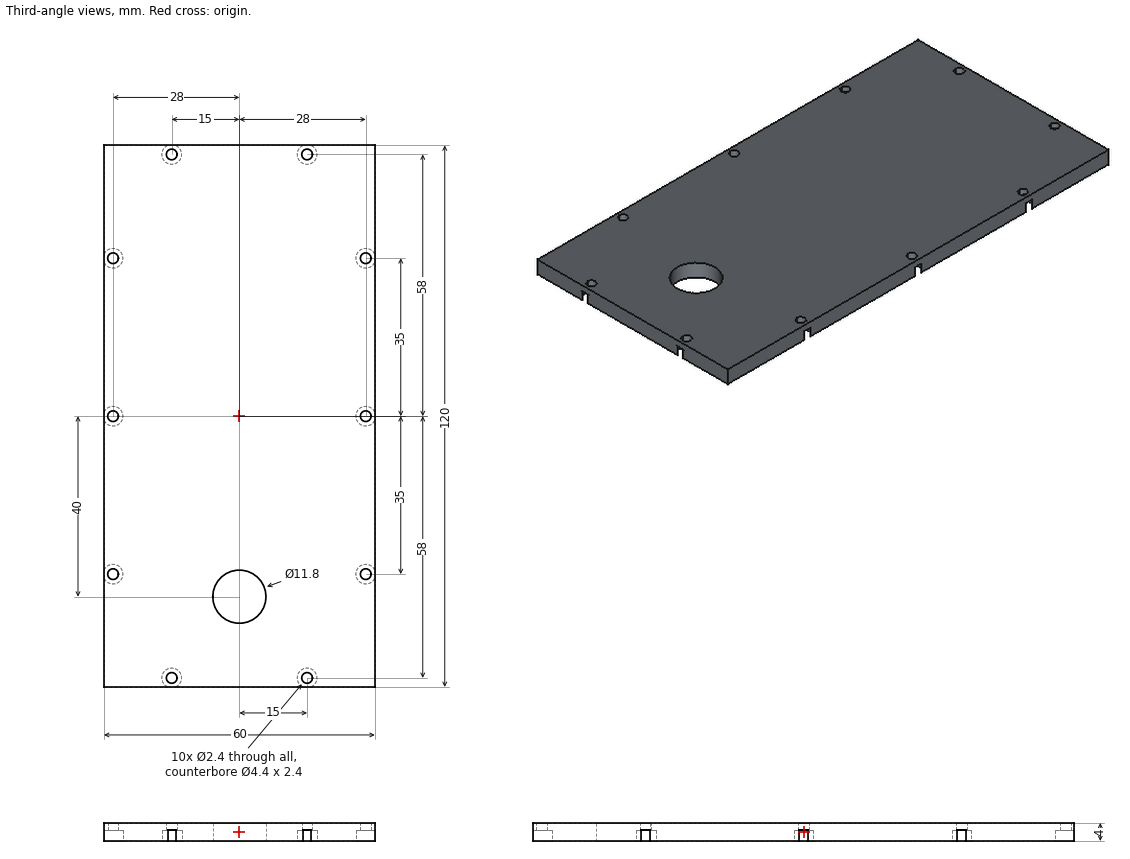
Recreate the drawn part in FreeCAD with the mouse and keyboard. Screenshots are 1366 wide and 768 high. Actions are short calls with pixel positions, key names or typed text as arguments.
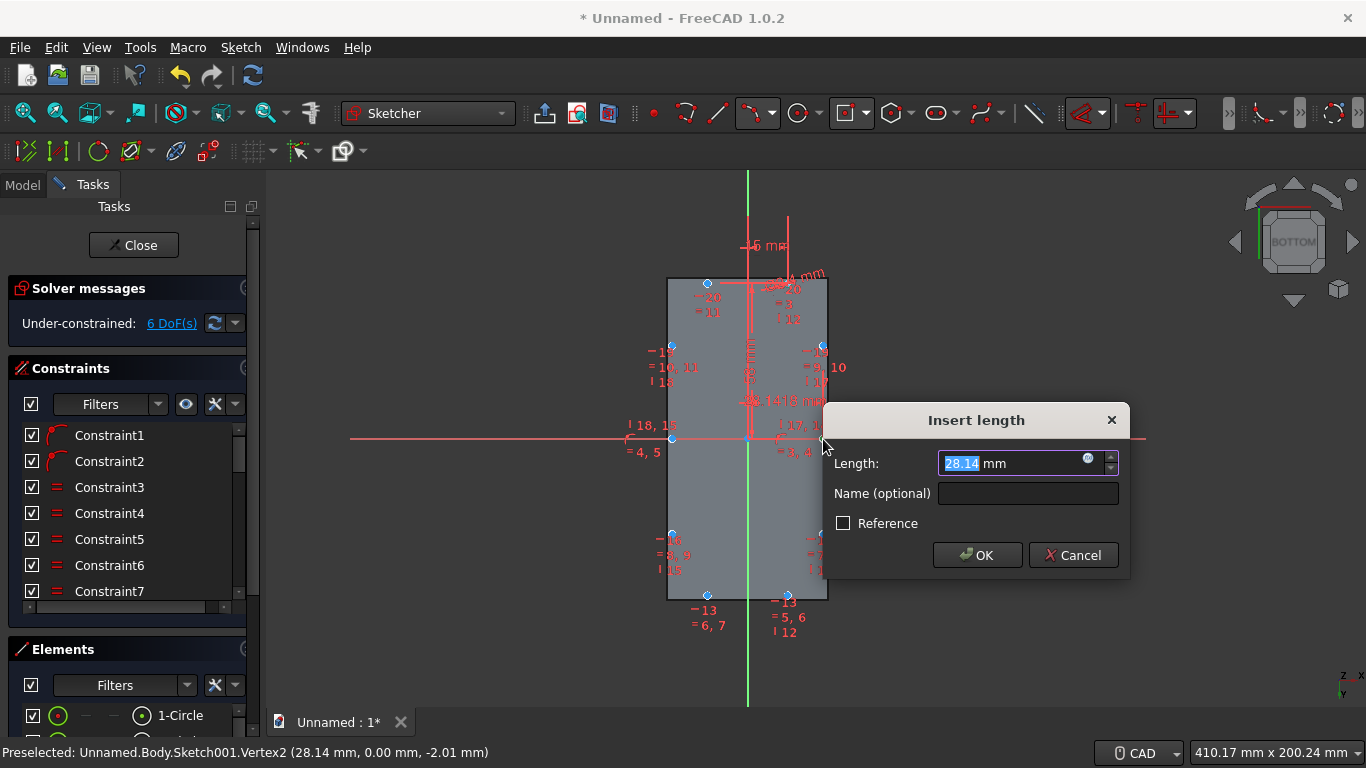
text(28)
key(Return)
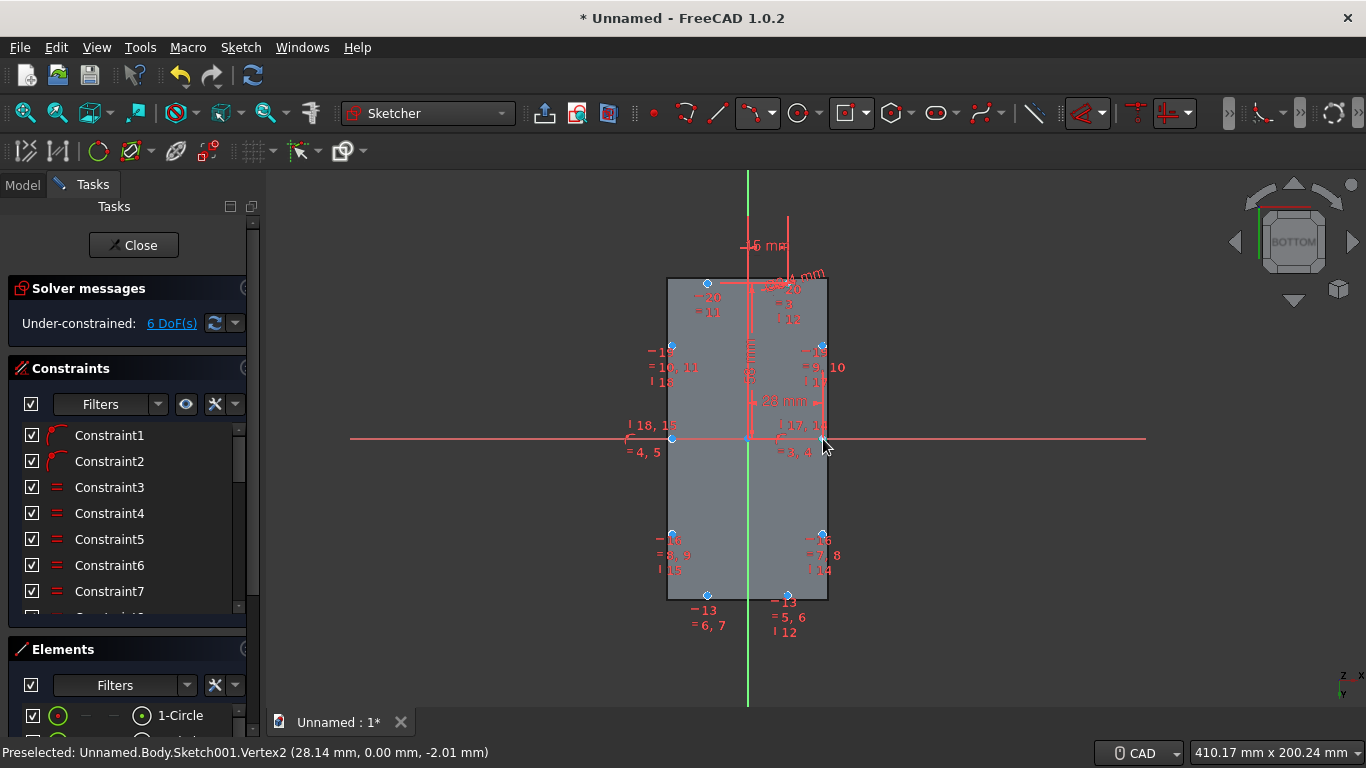
click(672, 439)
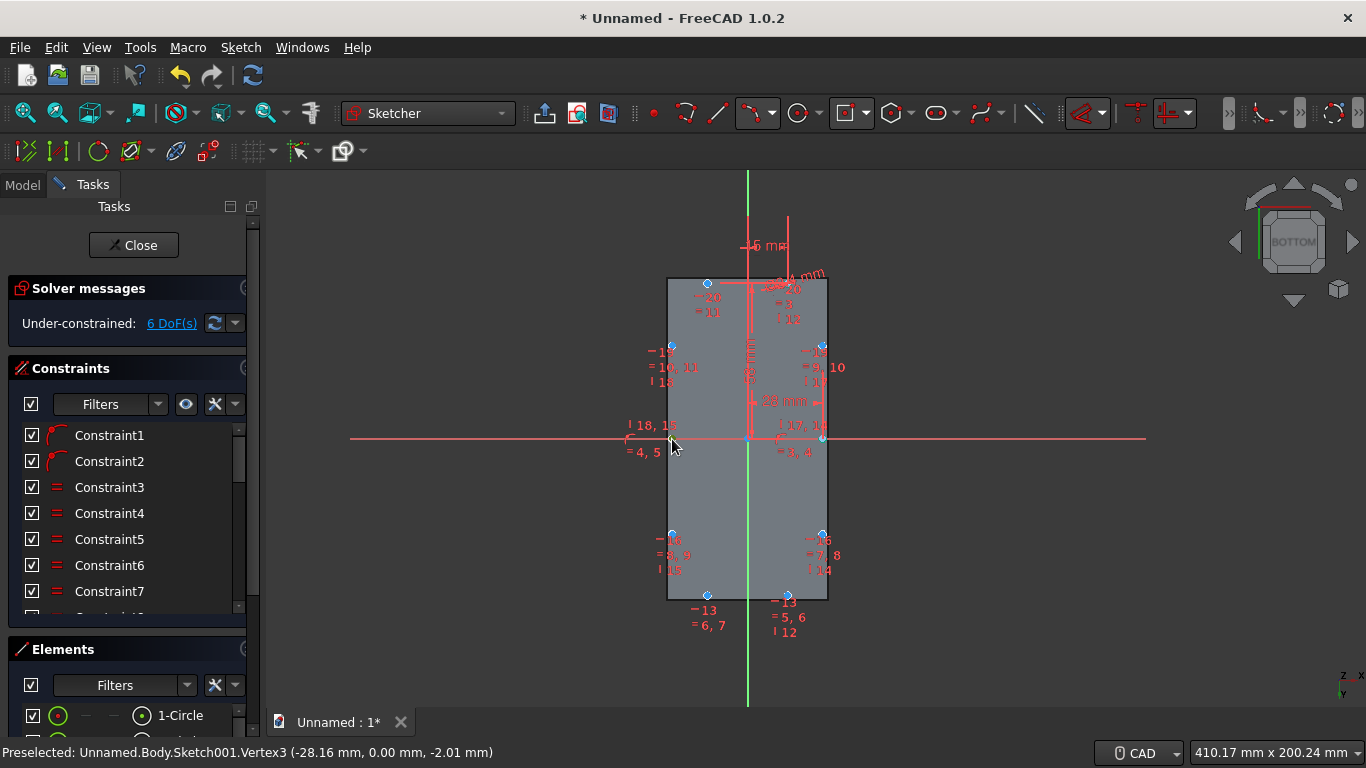
click(1104, 114)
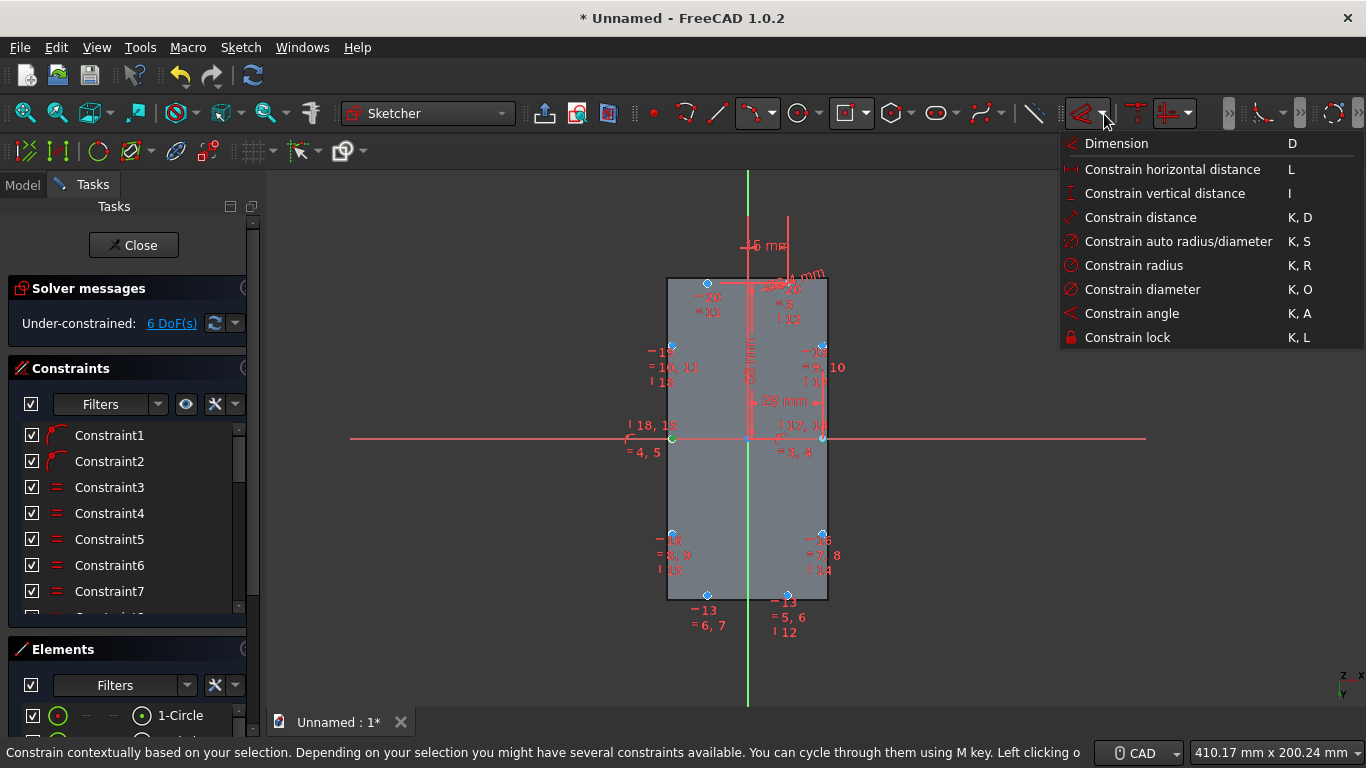
click(1212, 169)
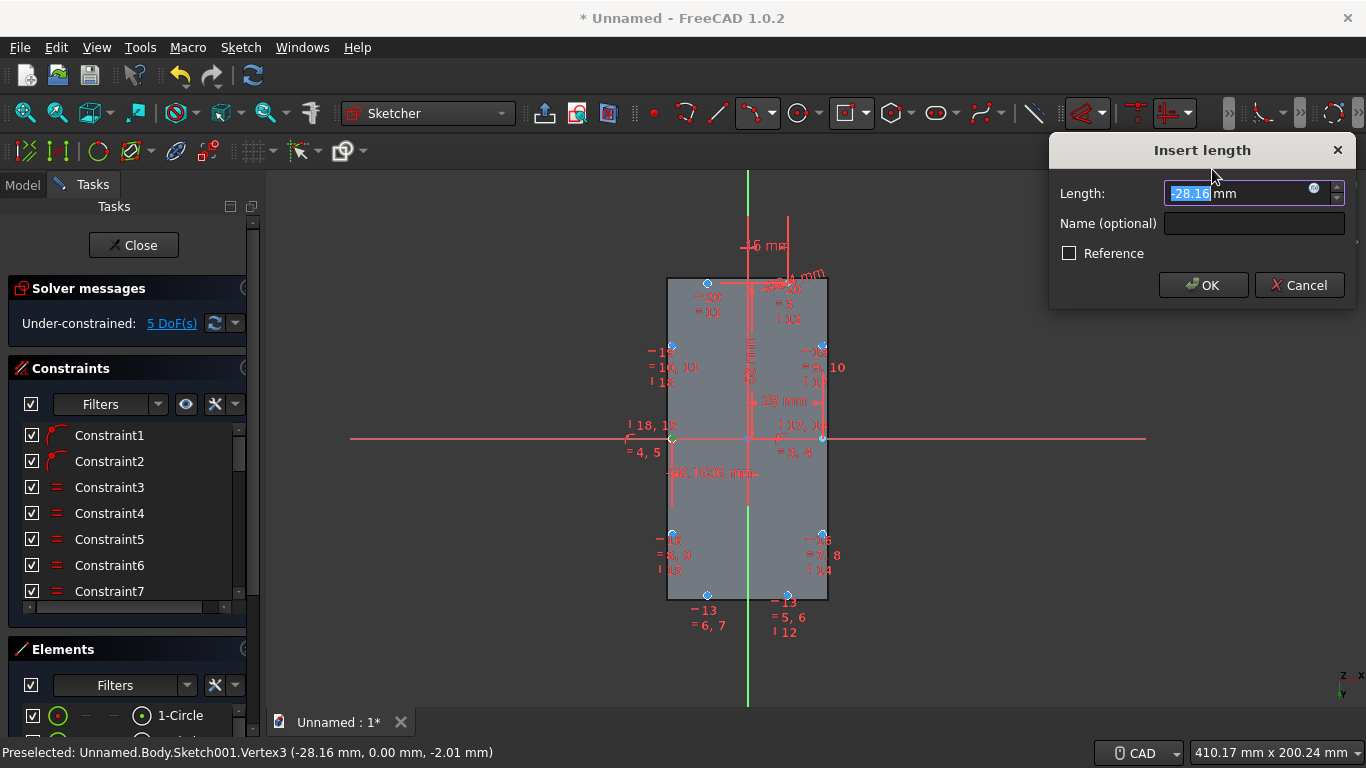
text(-28)
key(Return)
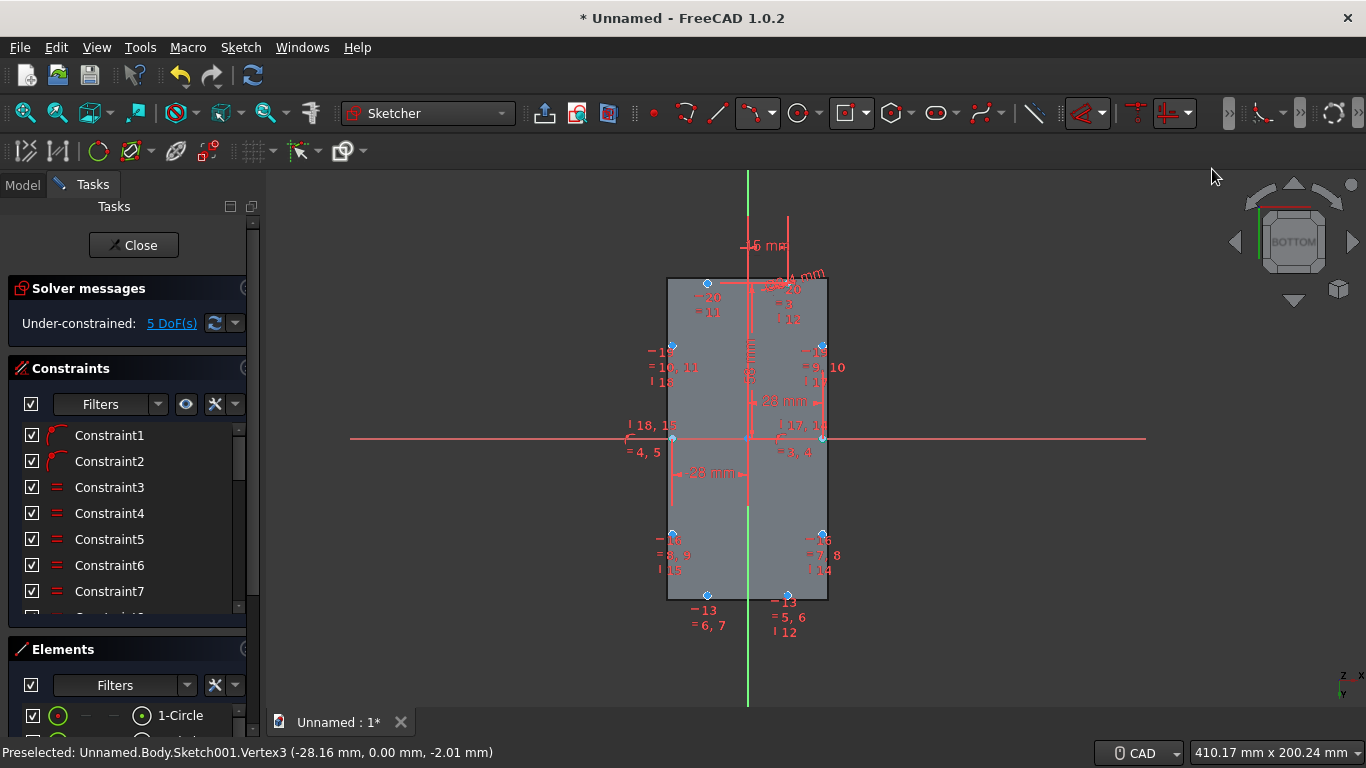
click(788, 596)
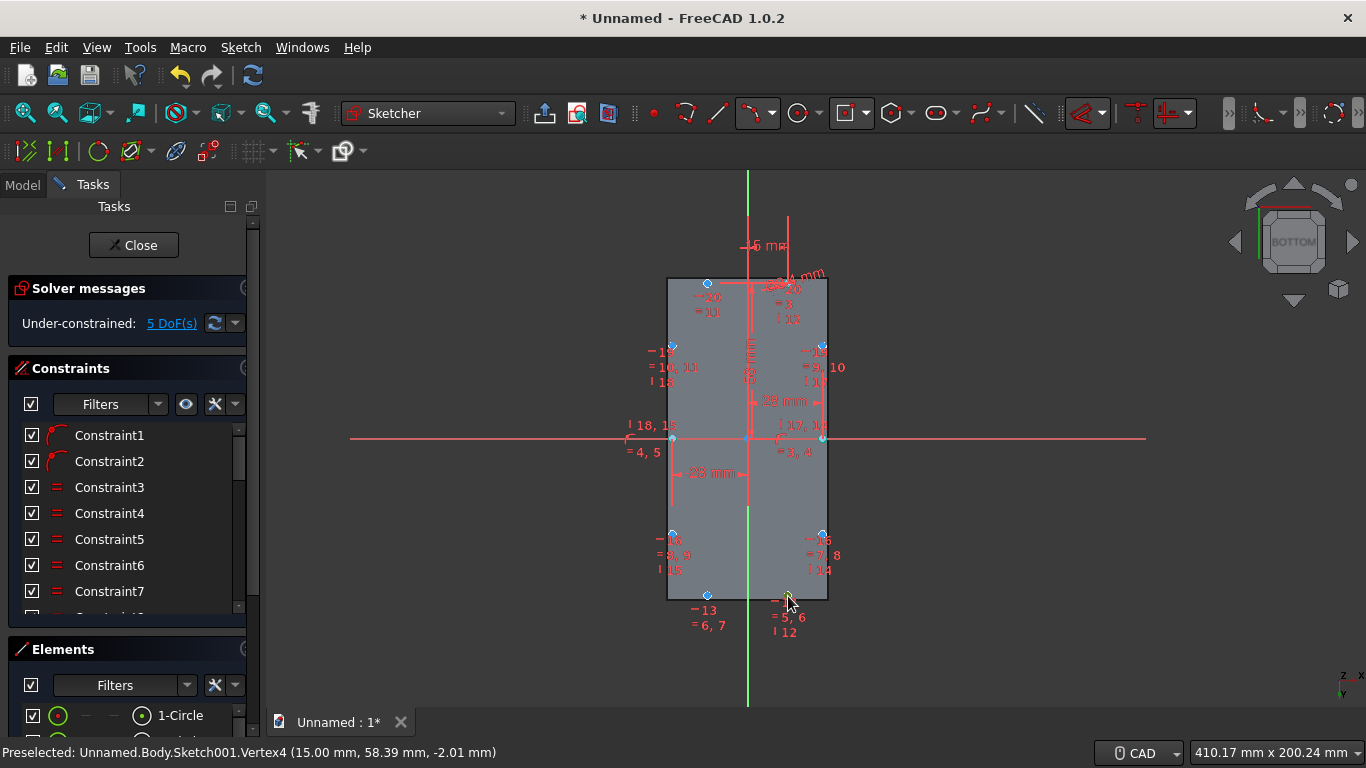
key(i)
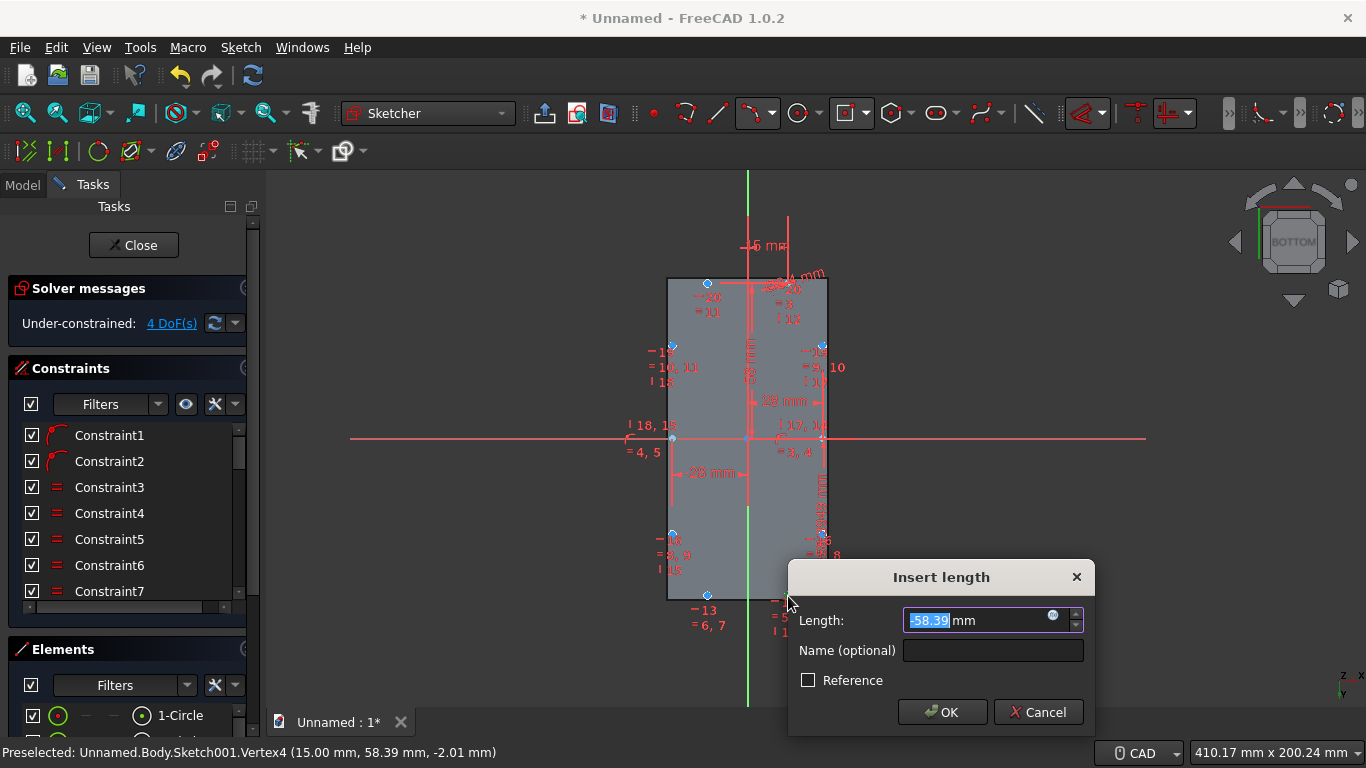
text(-58)
key(Return)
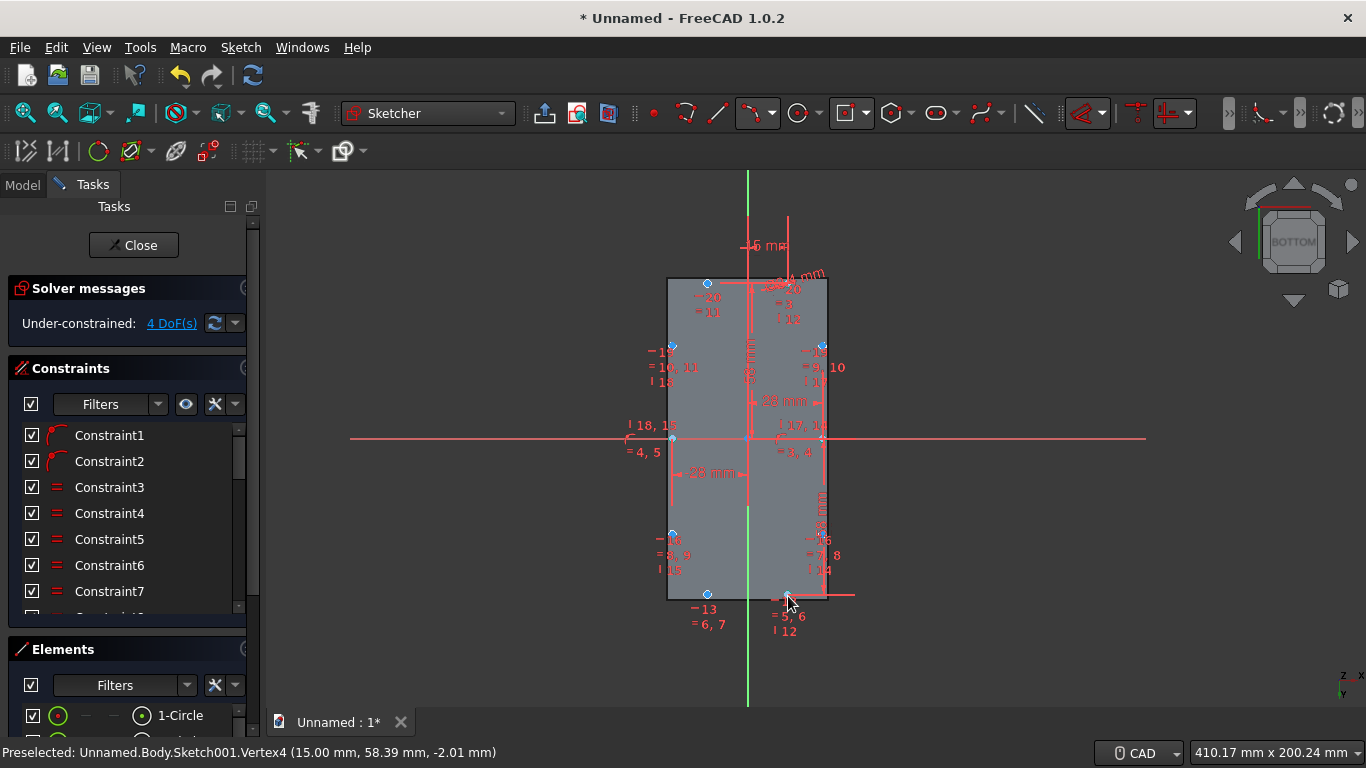
click(707, 595)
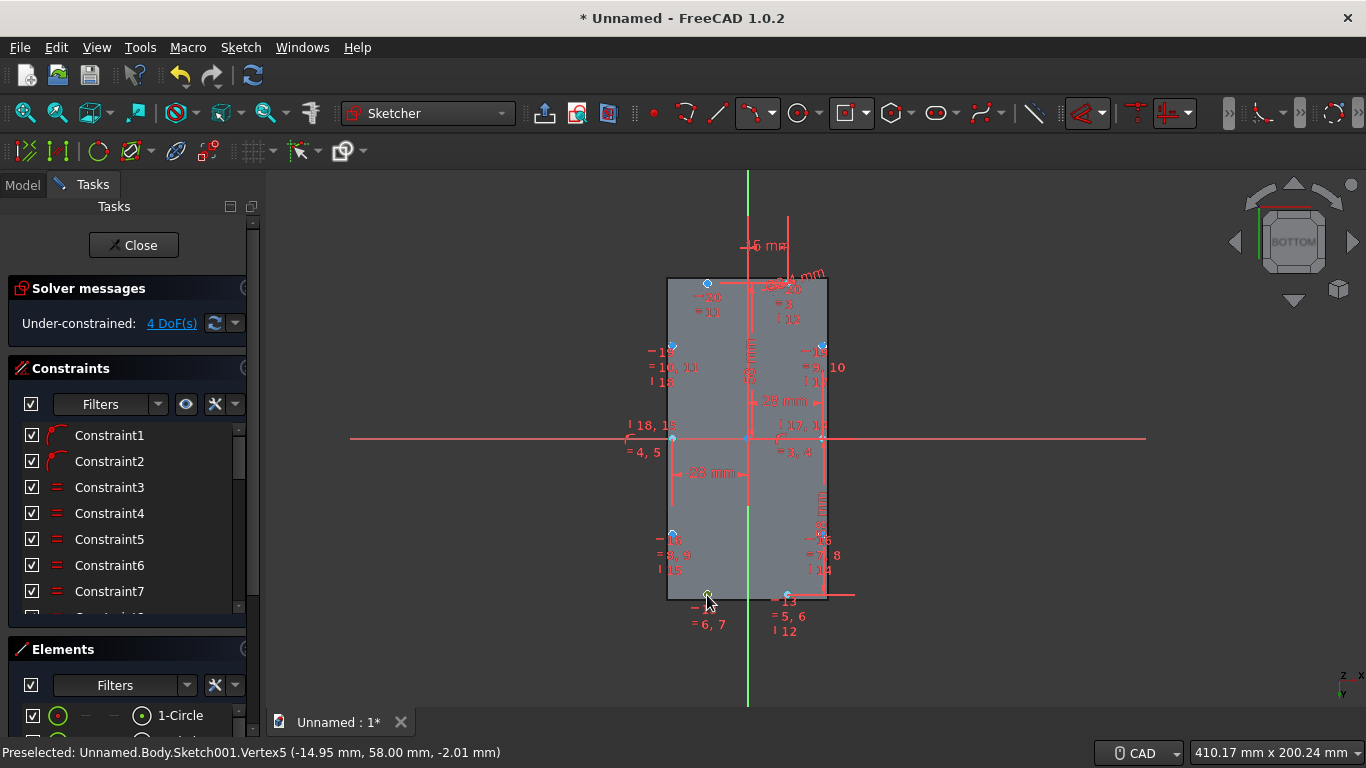
click(1104, 114)